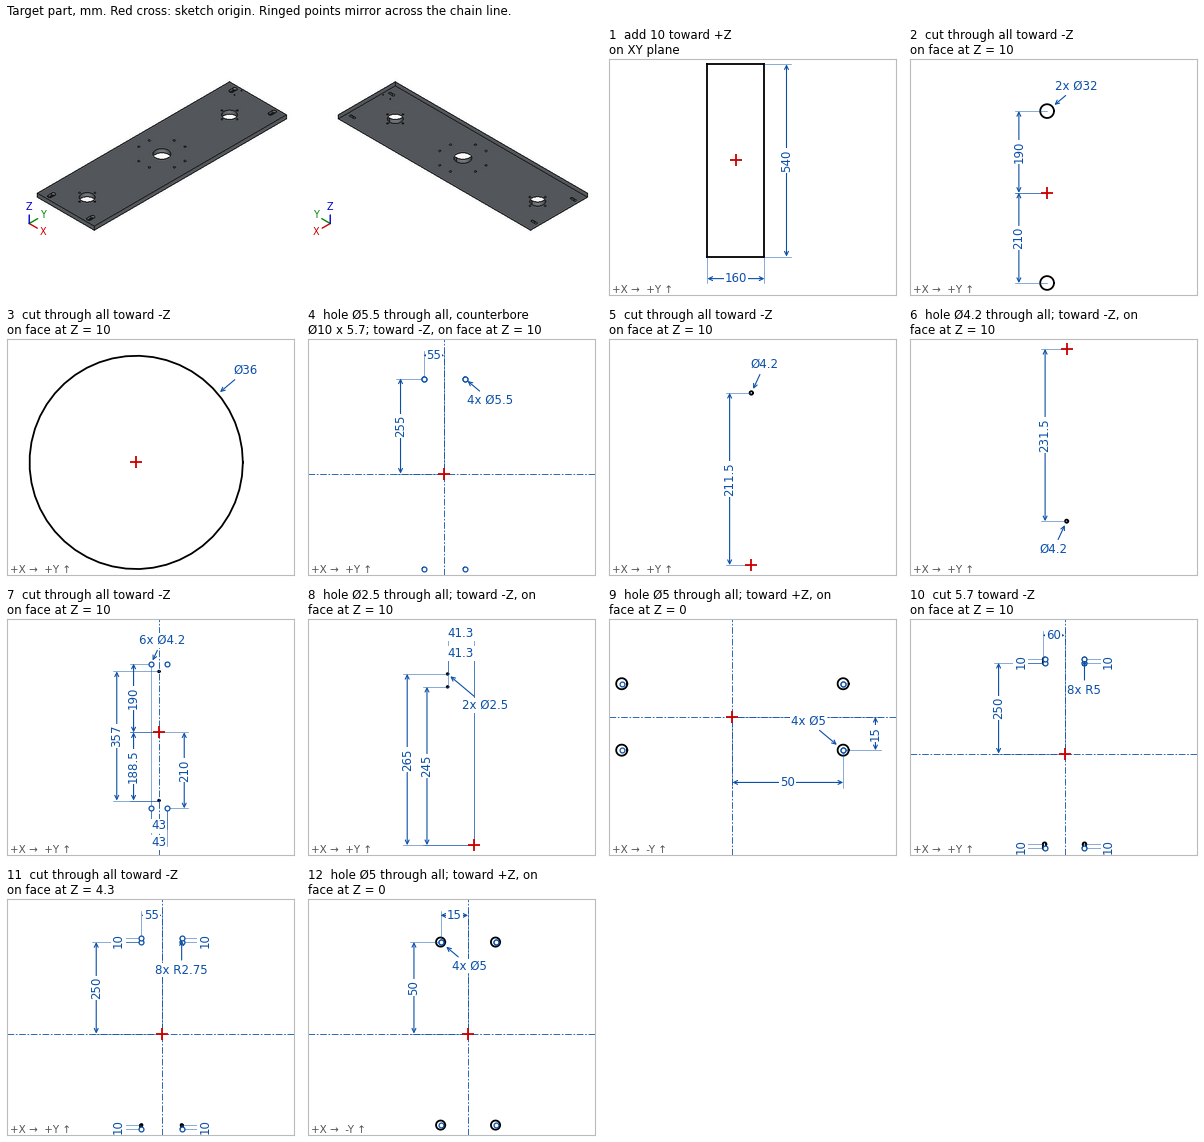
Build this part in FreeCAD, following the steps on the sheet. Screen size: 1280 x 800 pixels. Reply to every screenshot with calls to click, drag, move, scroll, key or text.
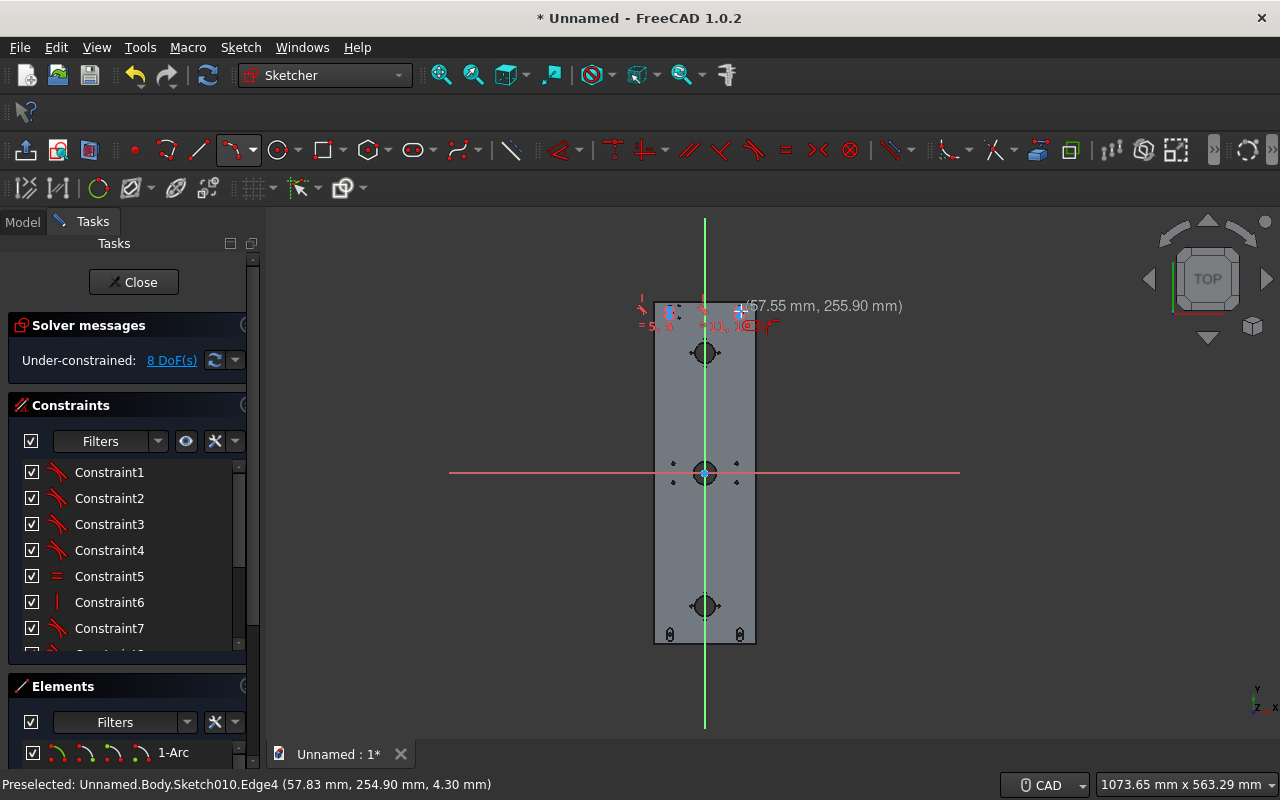
scroll(670, 638, up, 13)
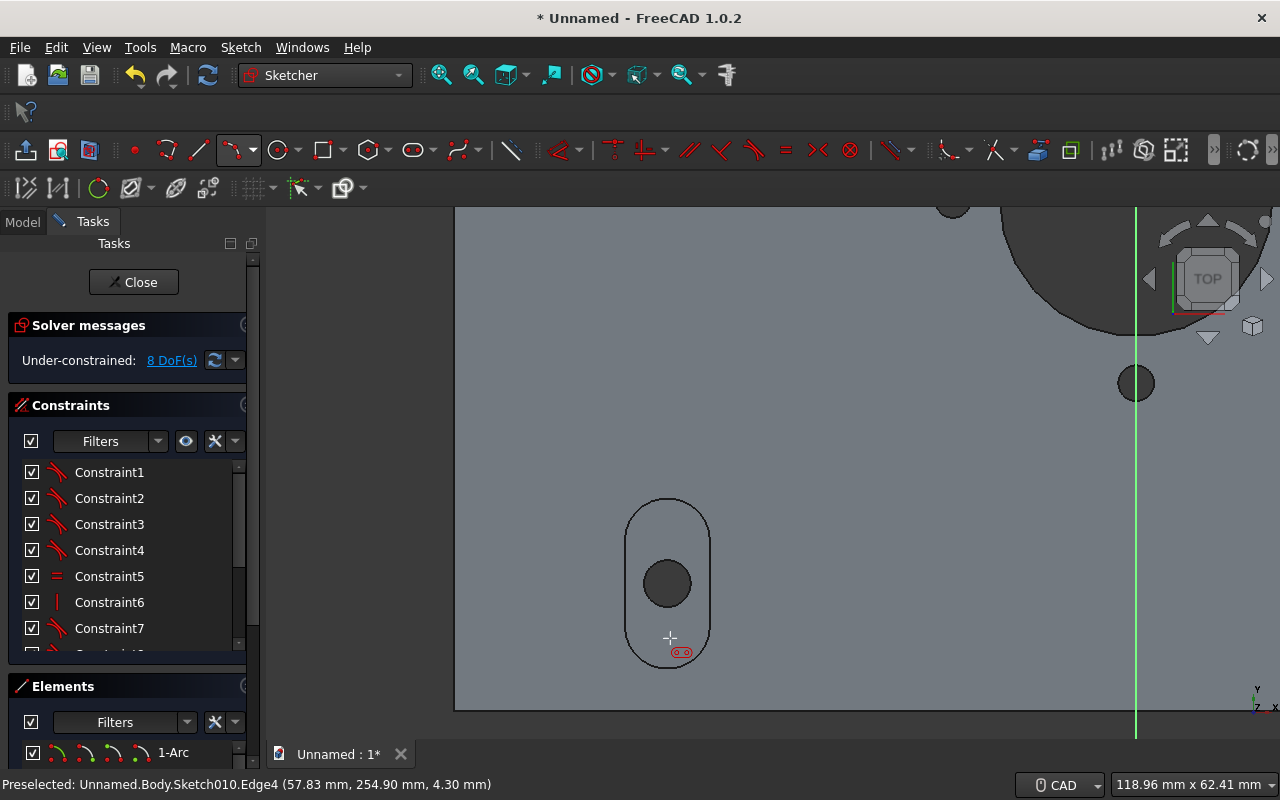
scroll(670, 639, down, 13)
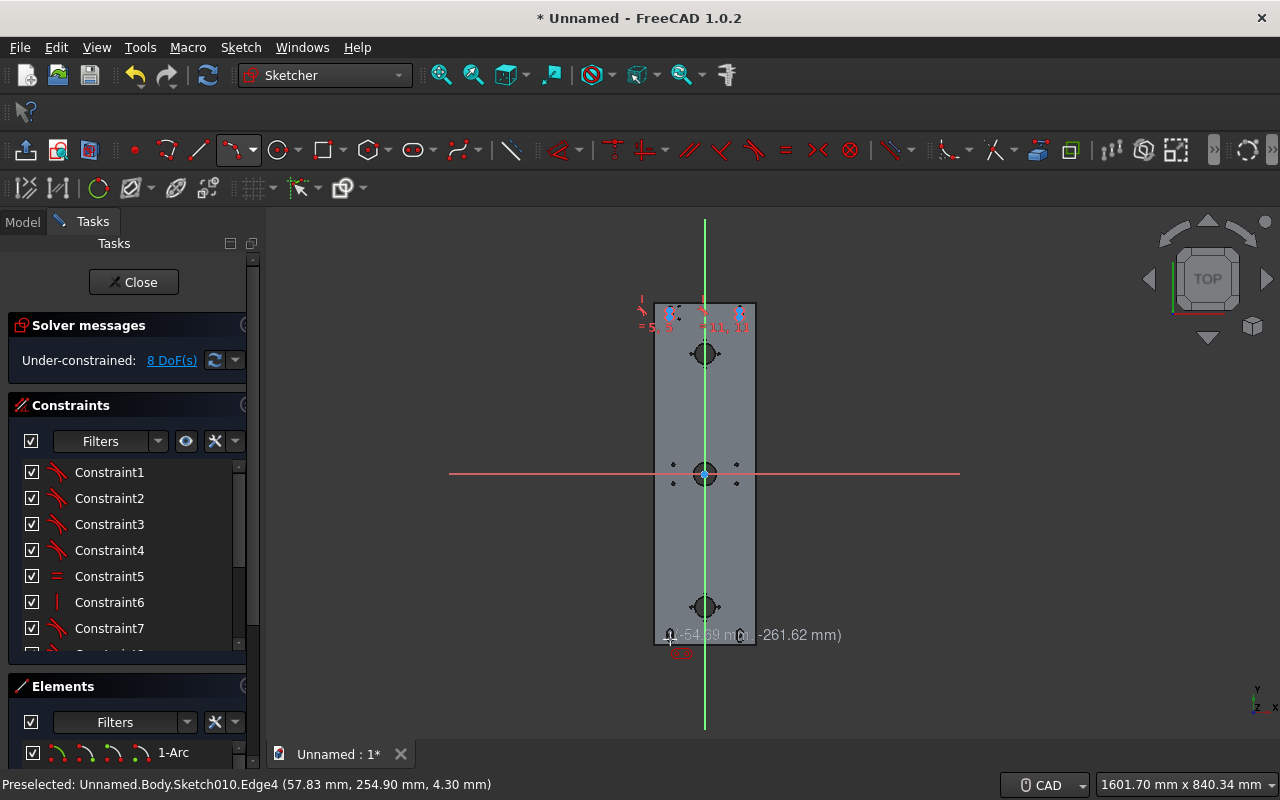
click(670, 639)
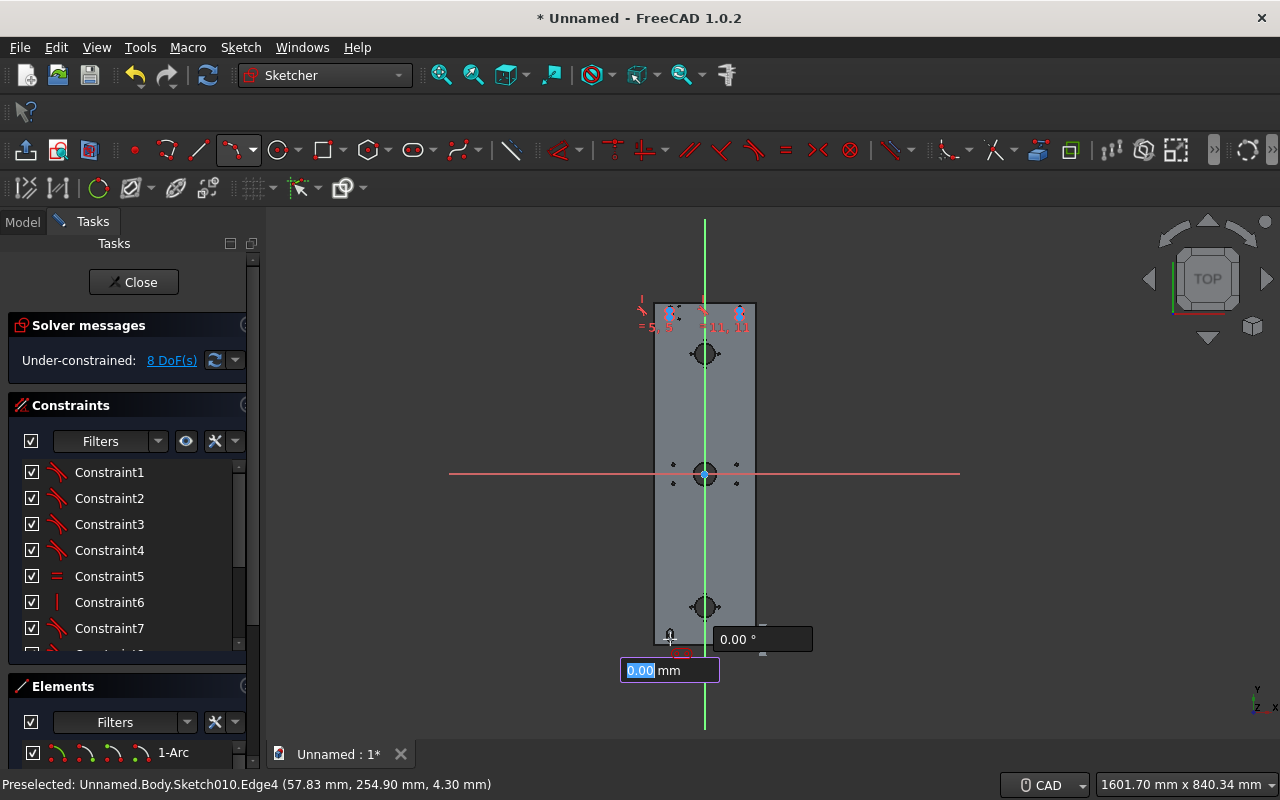
scroll(670, 632, up, 5)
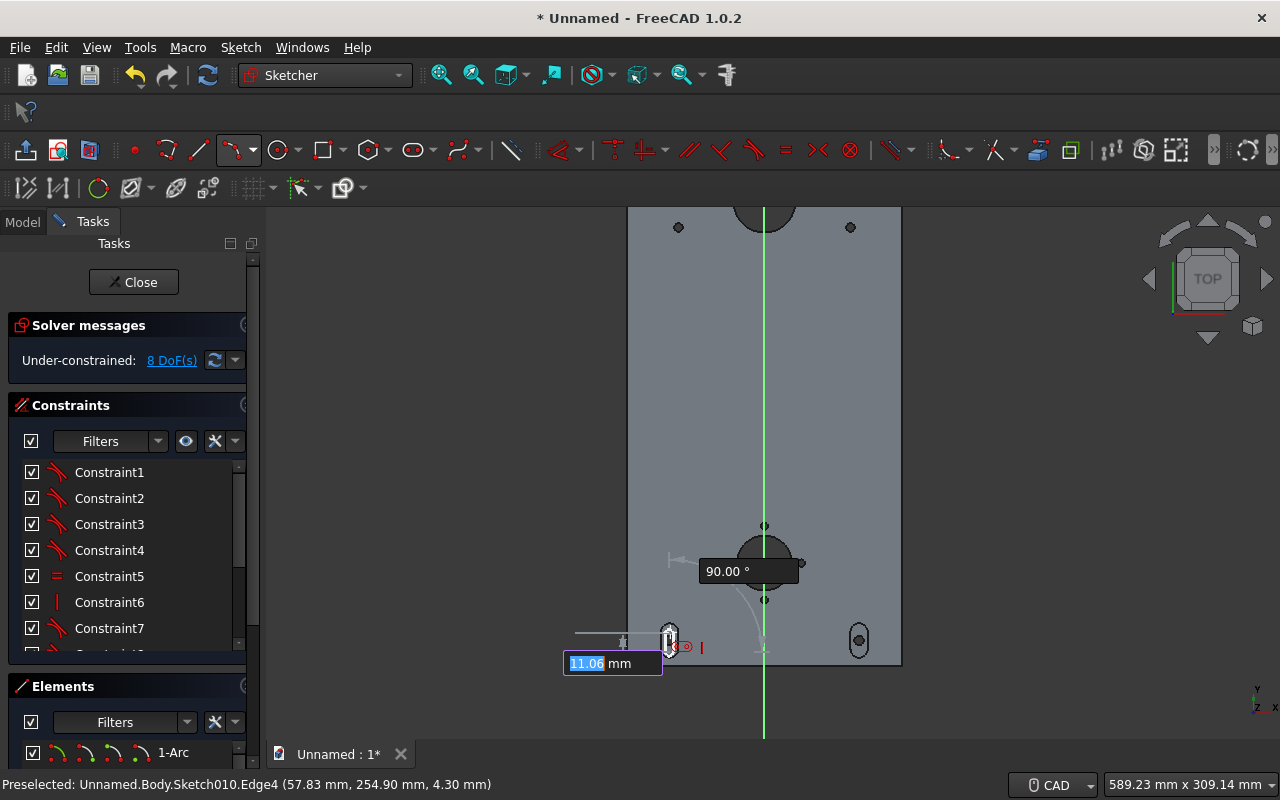
click(669, 632)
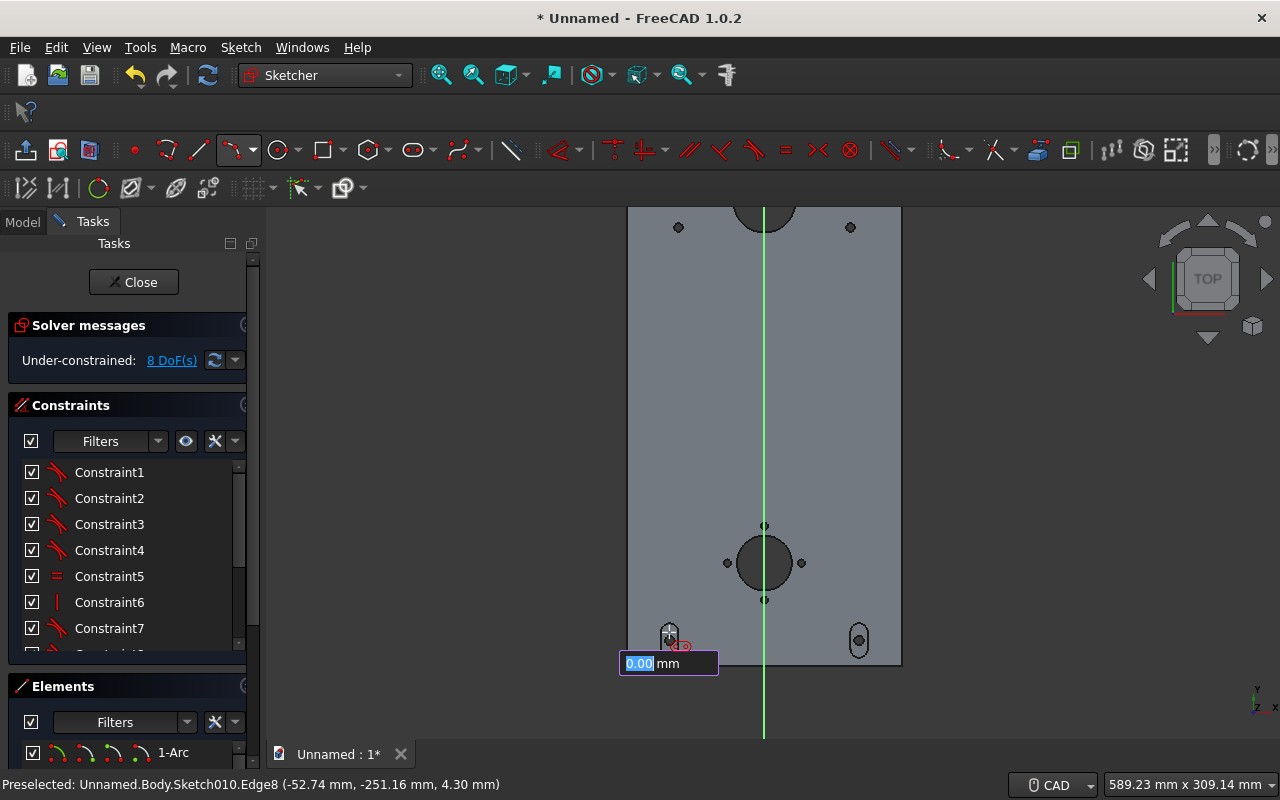
scroll(675, 641, up, 7)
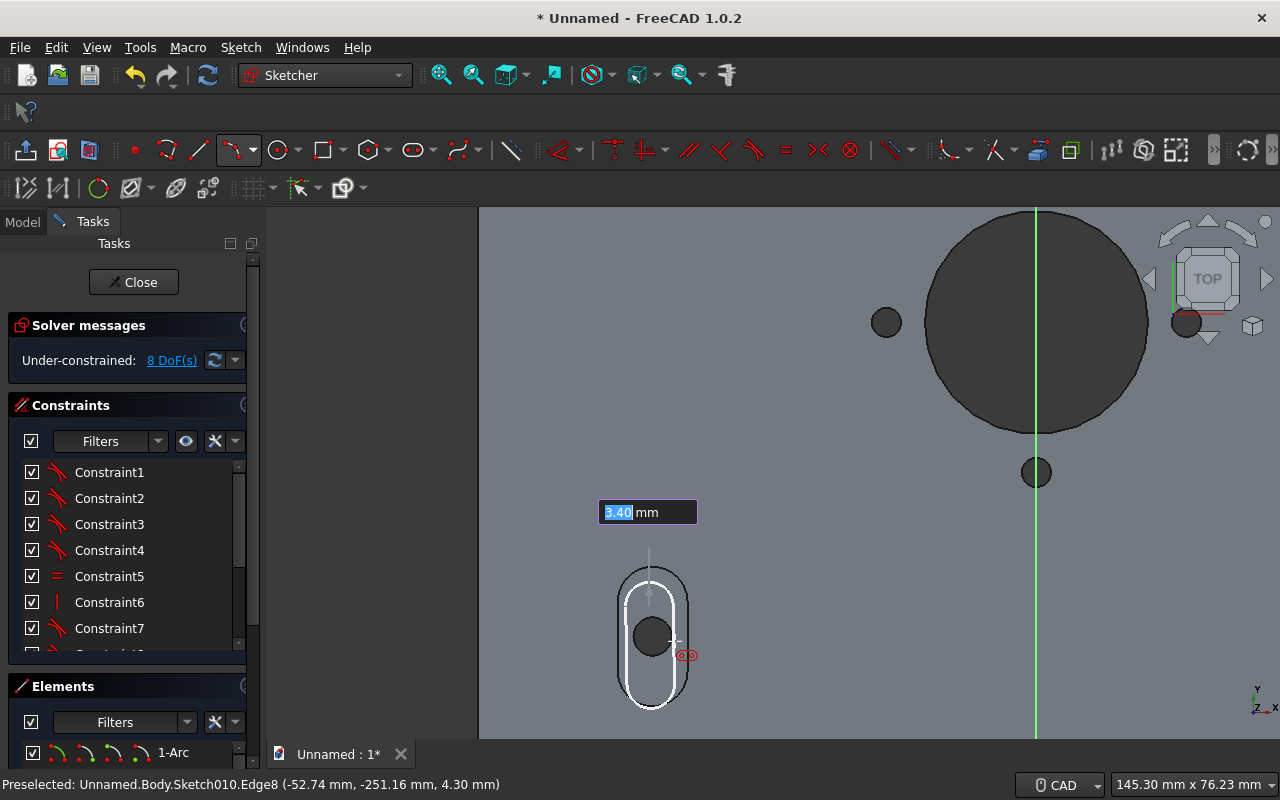
click(672, 637)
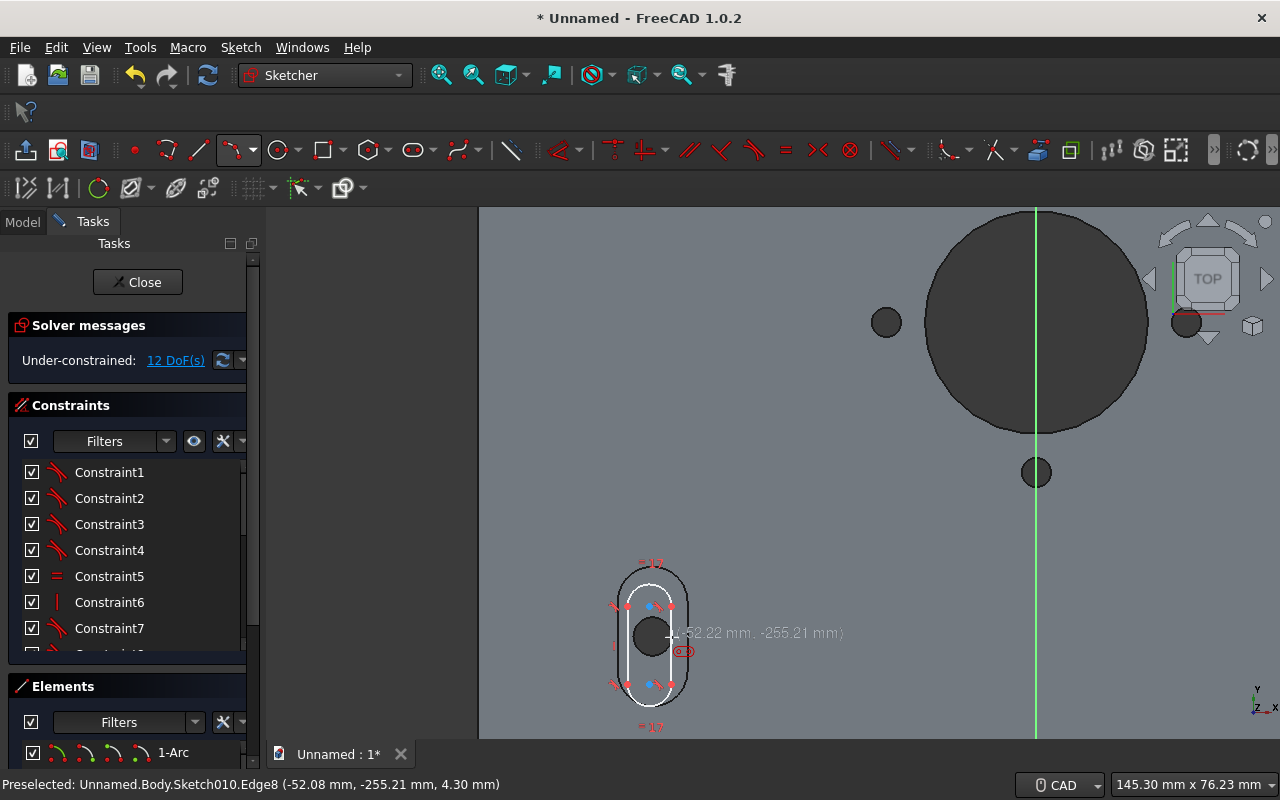
scroll(671, 634, down, 12)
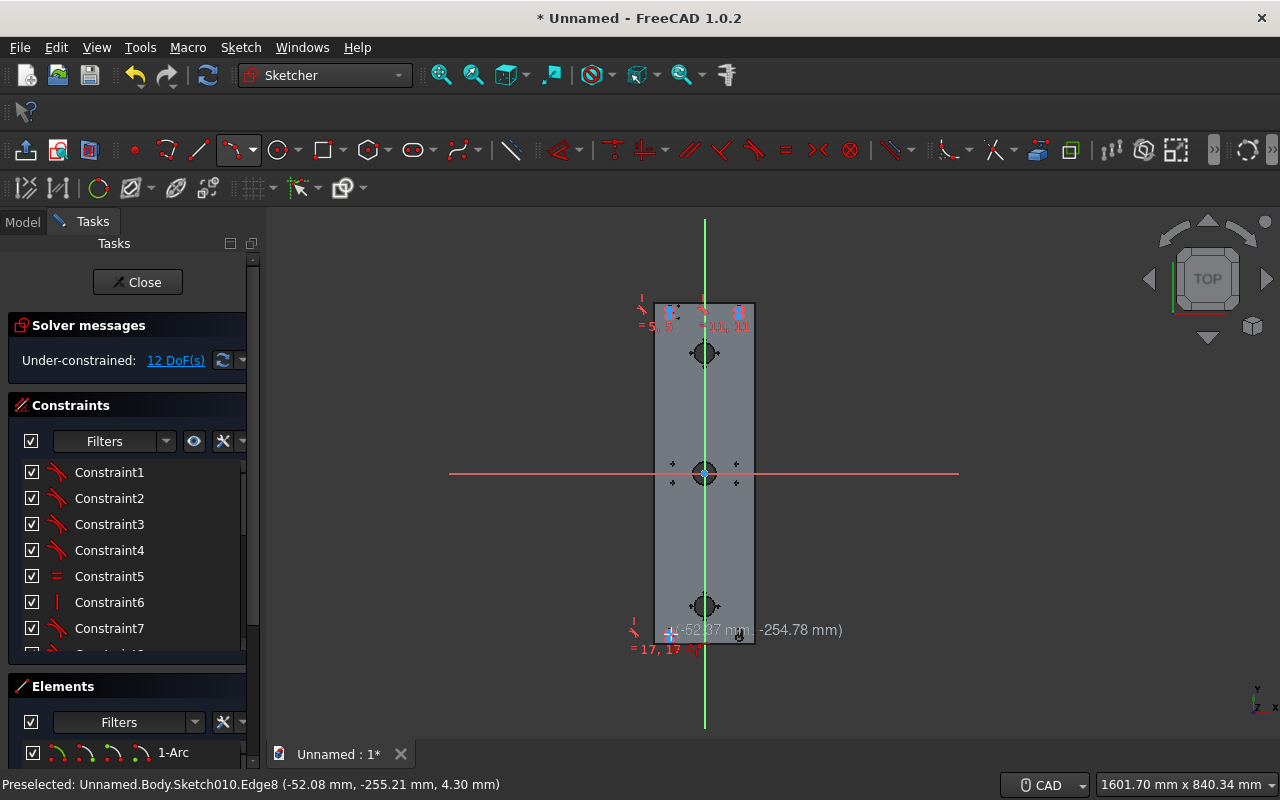
scroll(739, 638, up, 13)